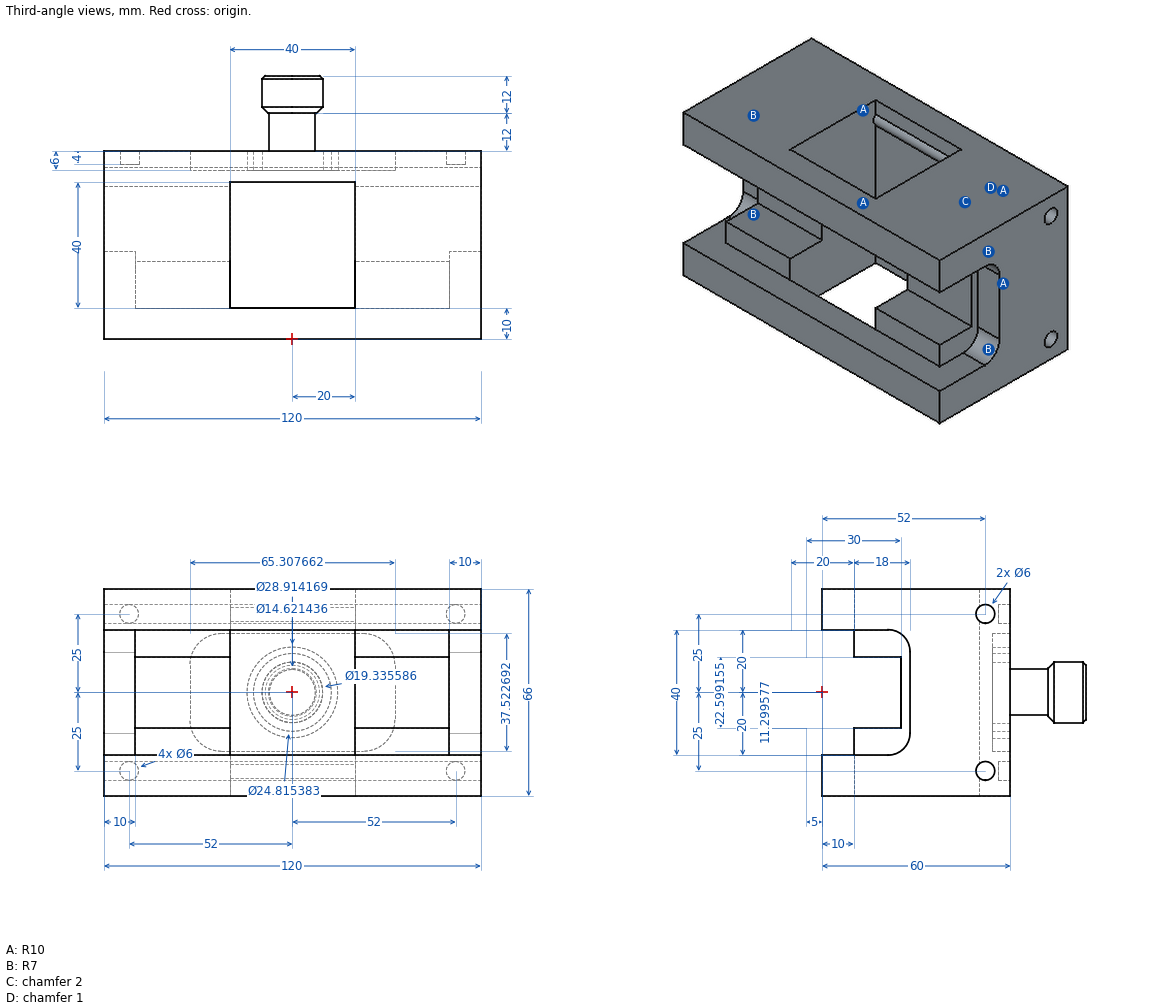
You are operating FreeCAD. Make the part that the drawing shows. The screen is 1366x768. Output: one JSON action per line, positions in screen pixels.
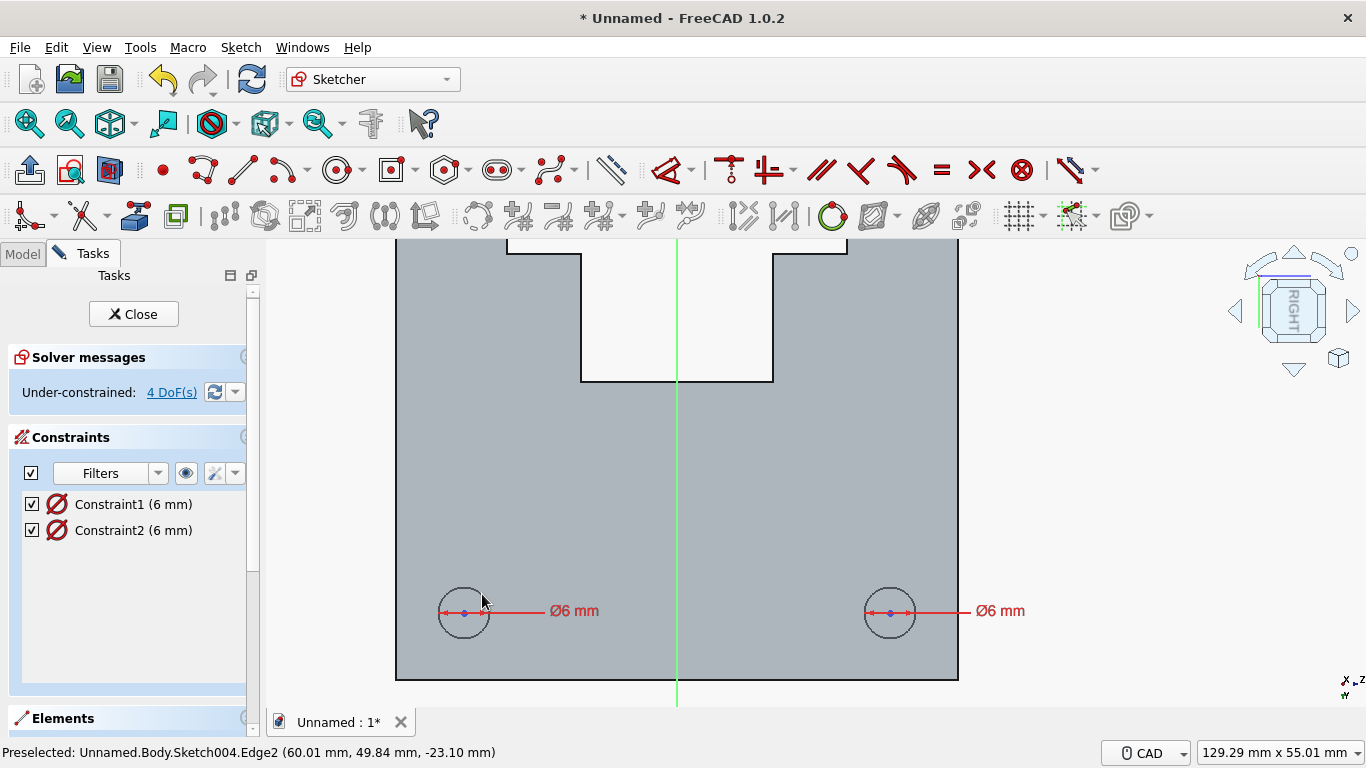
{"action": "left_click", "coordinate": [890, 613]}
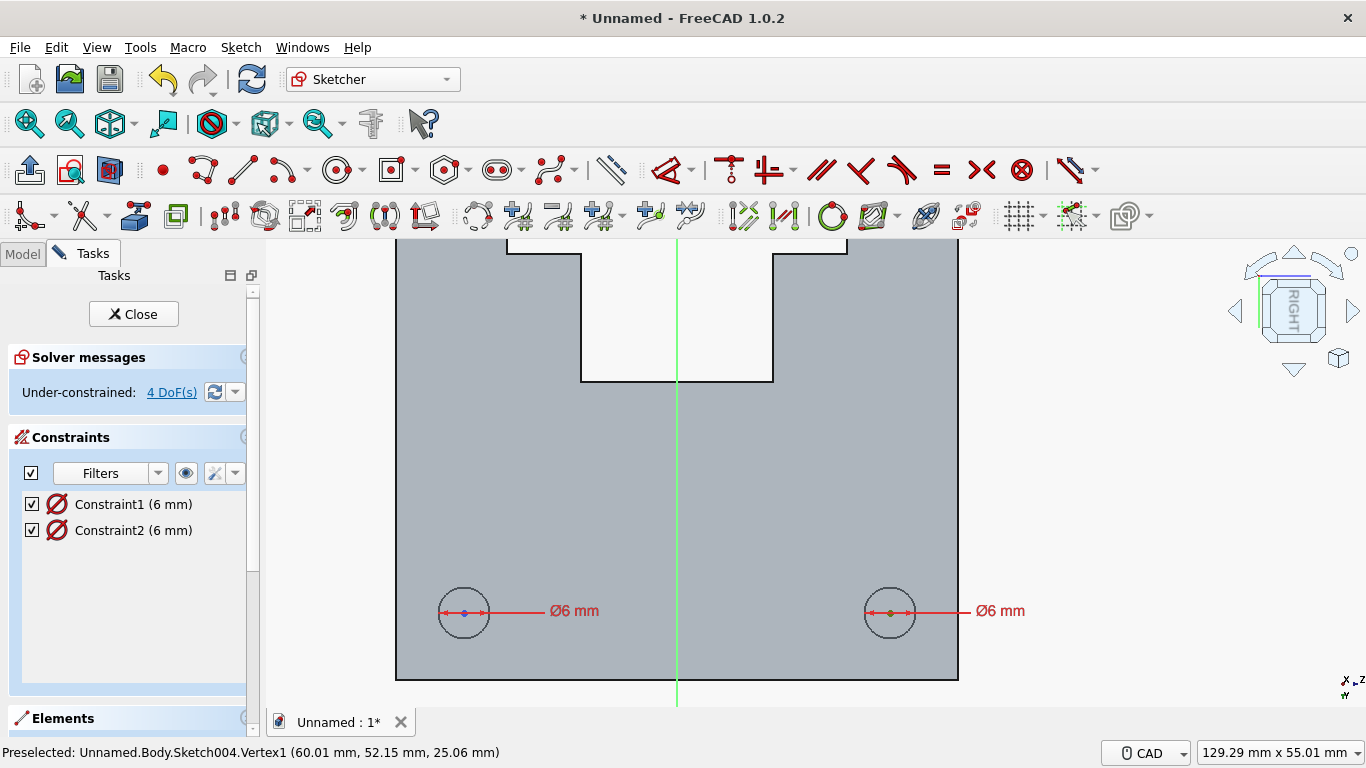
{"action": "left_click", "coordinate": [464, 613]}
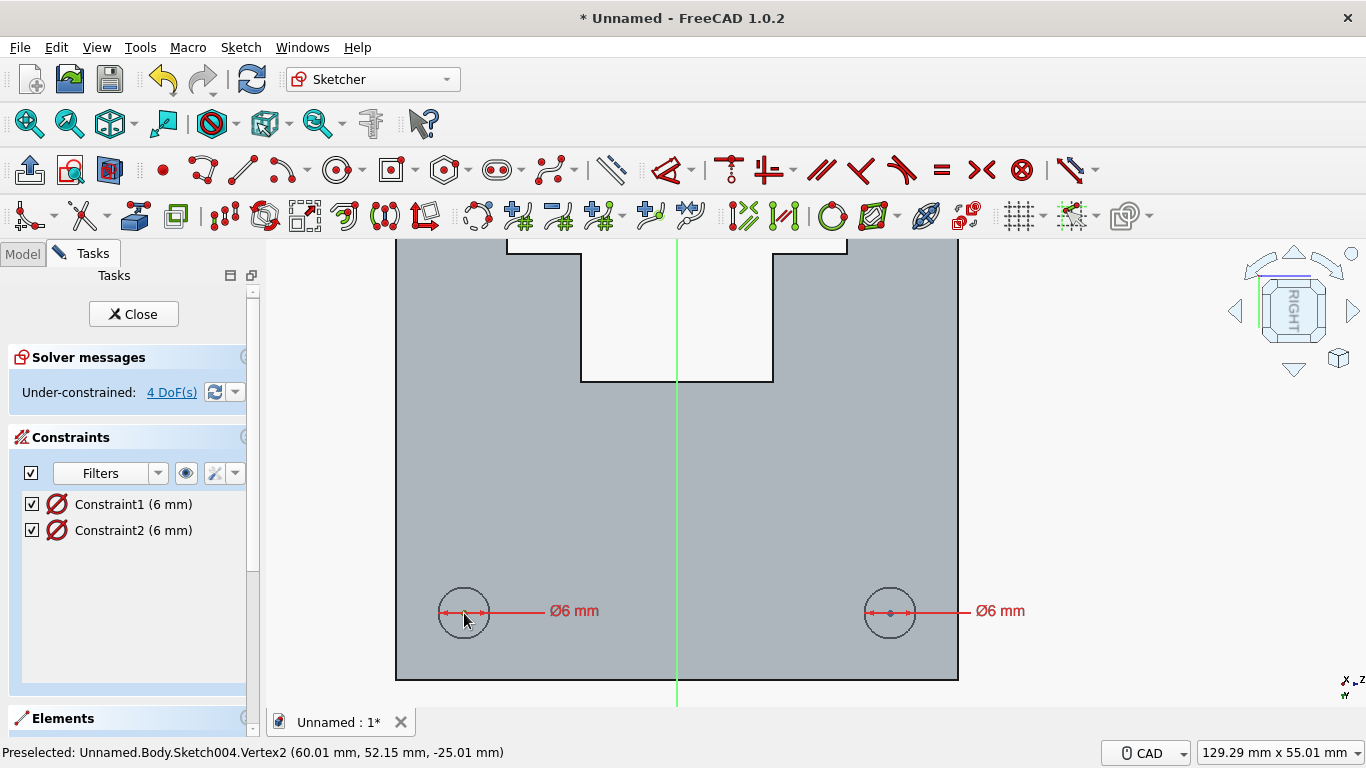
{"action": "key", "text": "h"}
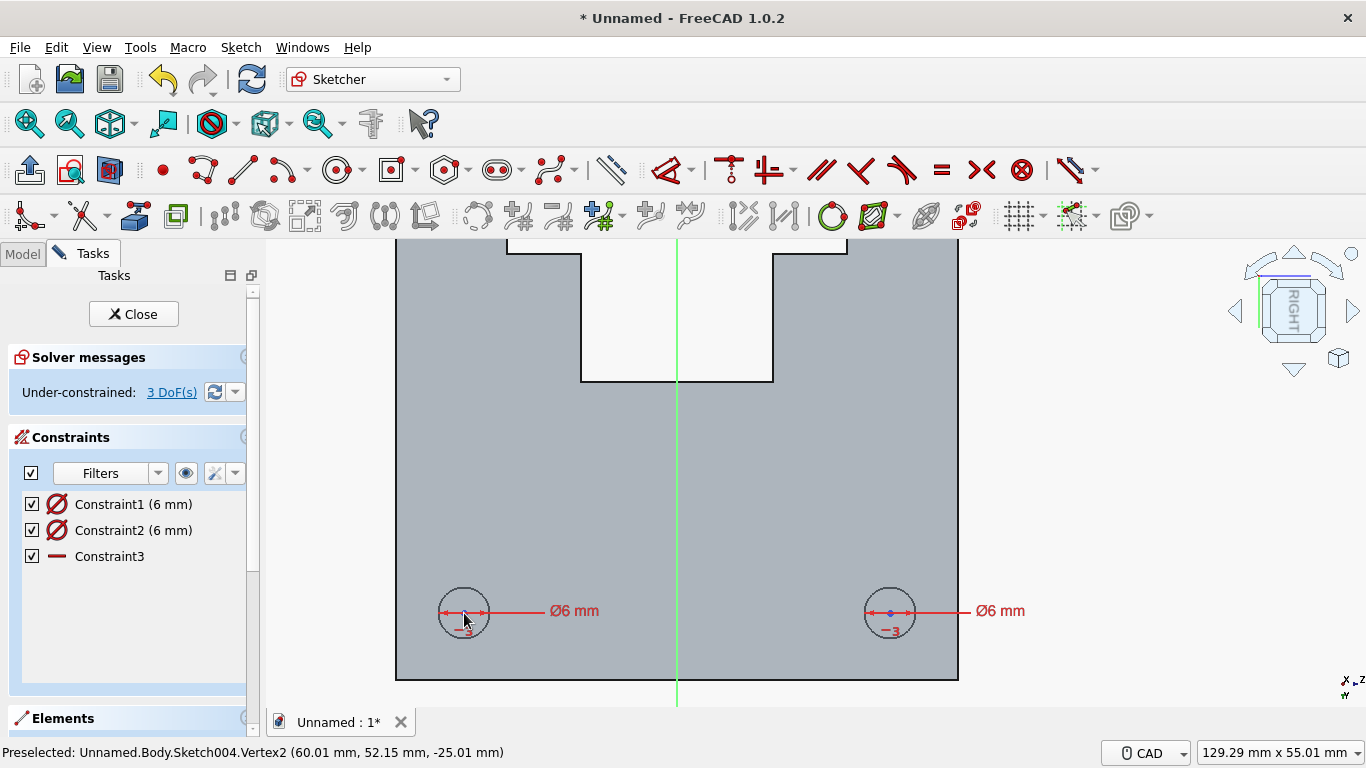
{"action": "left_click", "coordinate": [666, 170]}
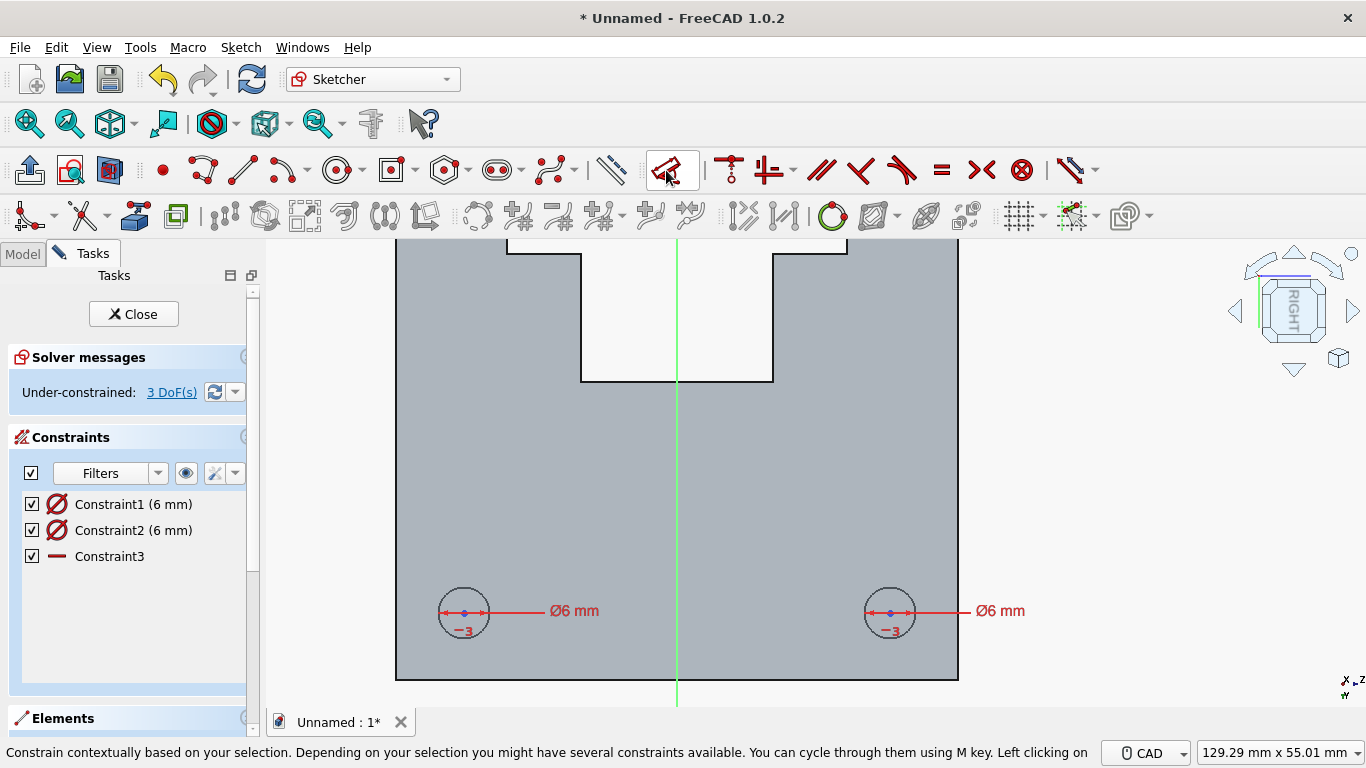
{"action": "left_click", "coordinate": [890, 613]}
{"action": "left_click", "coordinate": [783, 647]}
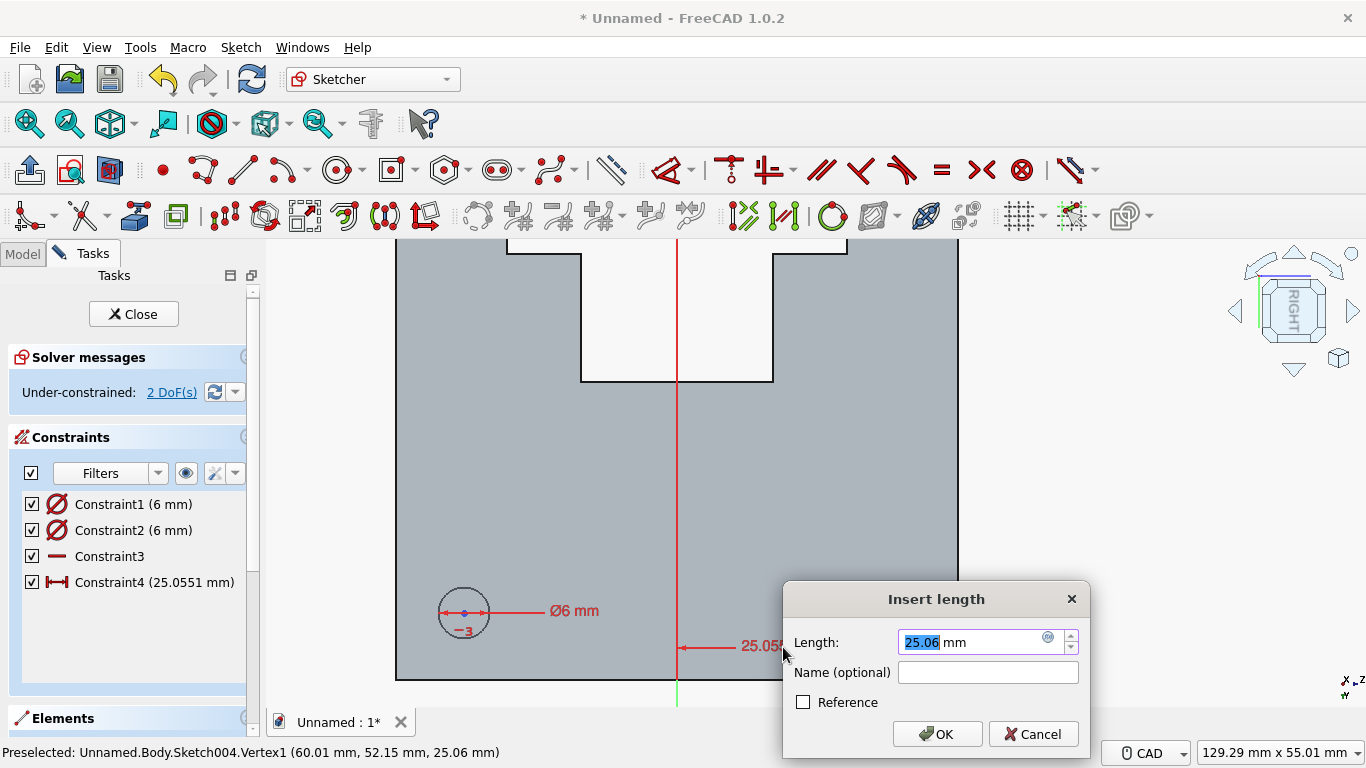
{"action": "type", "text": "25"}
{"action": "key", "text": "Return"}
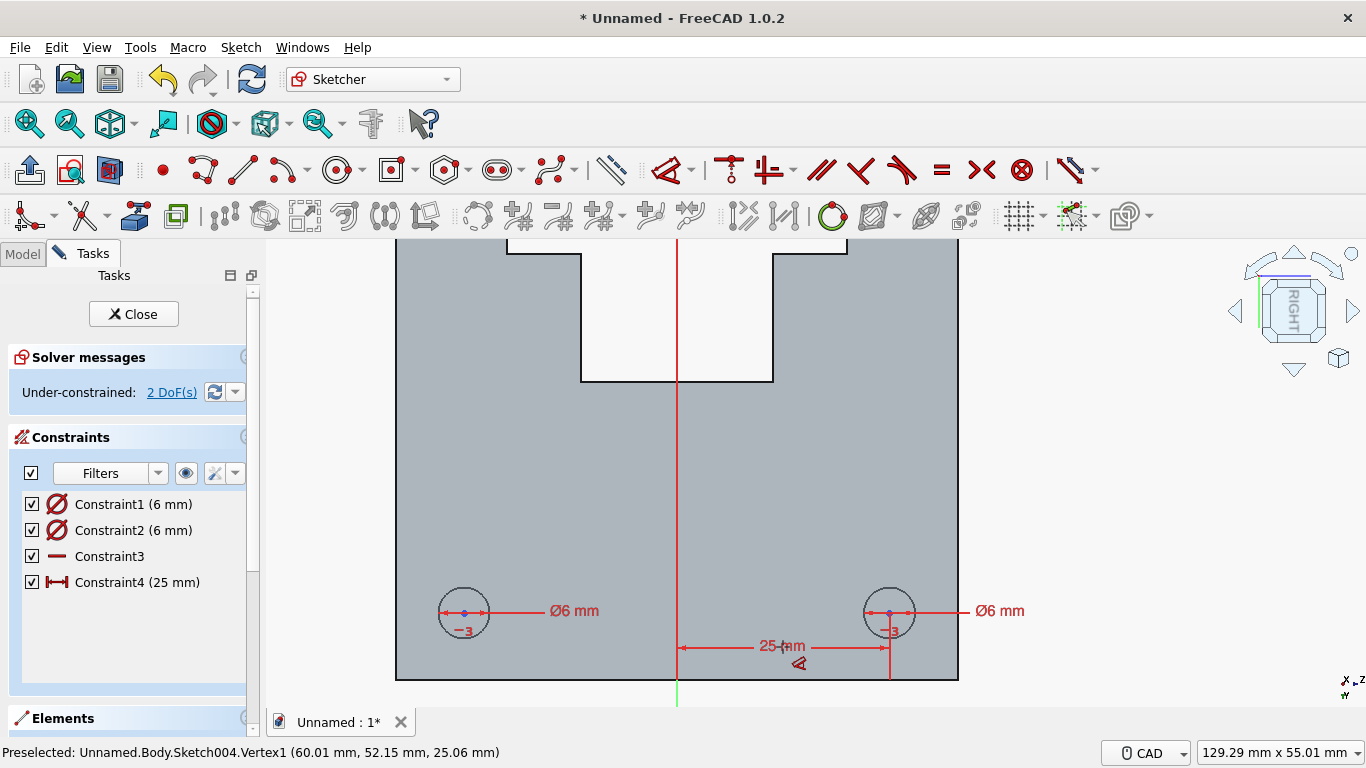
{"action": "left_click", "coordinate": [890, 613]}
{"action": "left_click", "coordinate": [924, 440]}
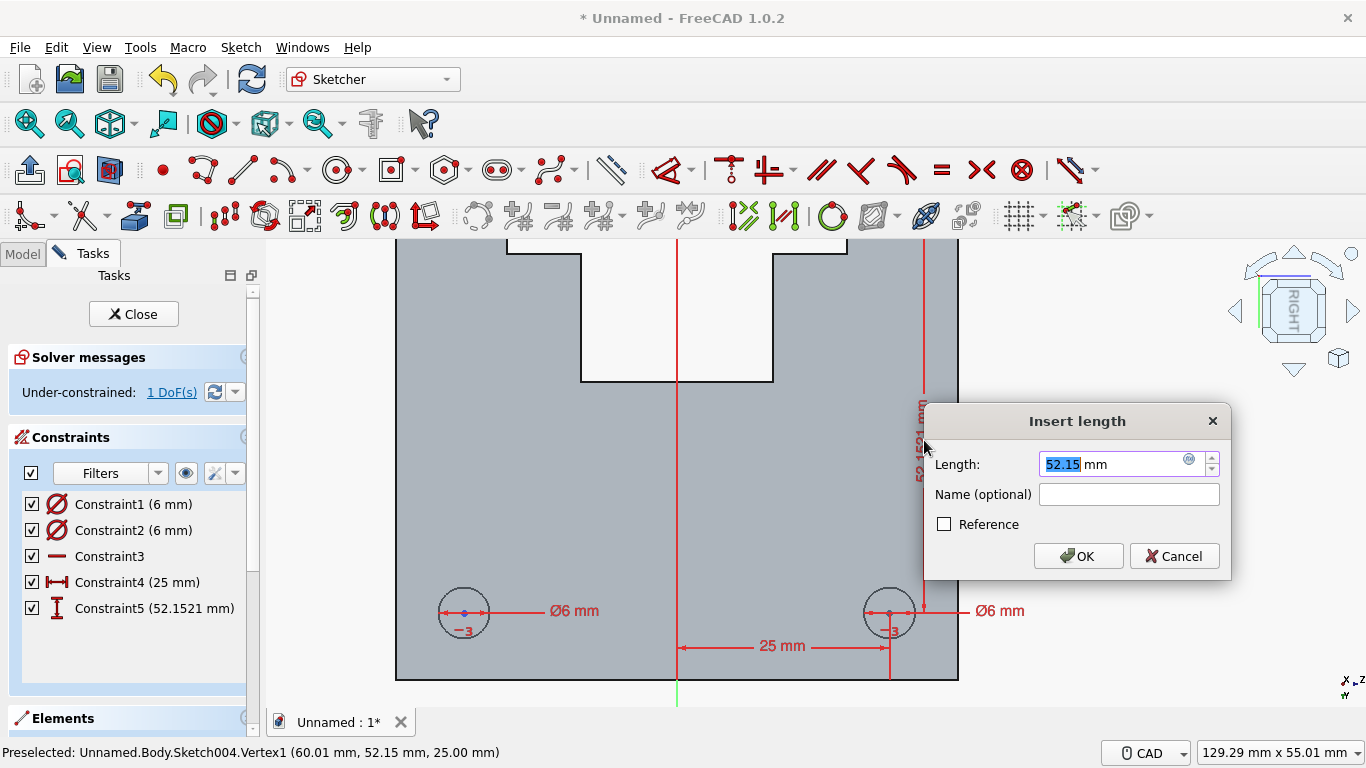
{"action": "type", "text": "52"}
{"action": "key", "text": "Return"}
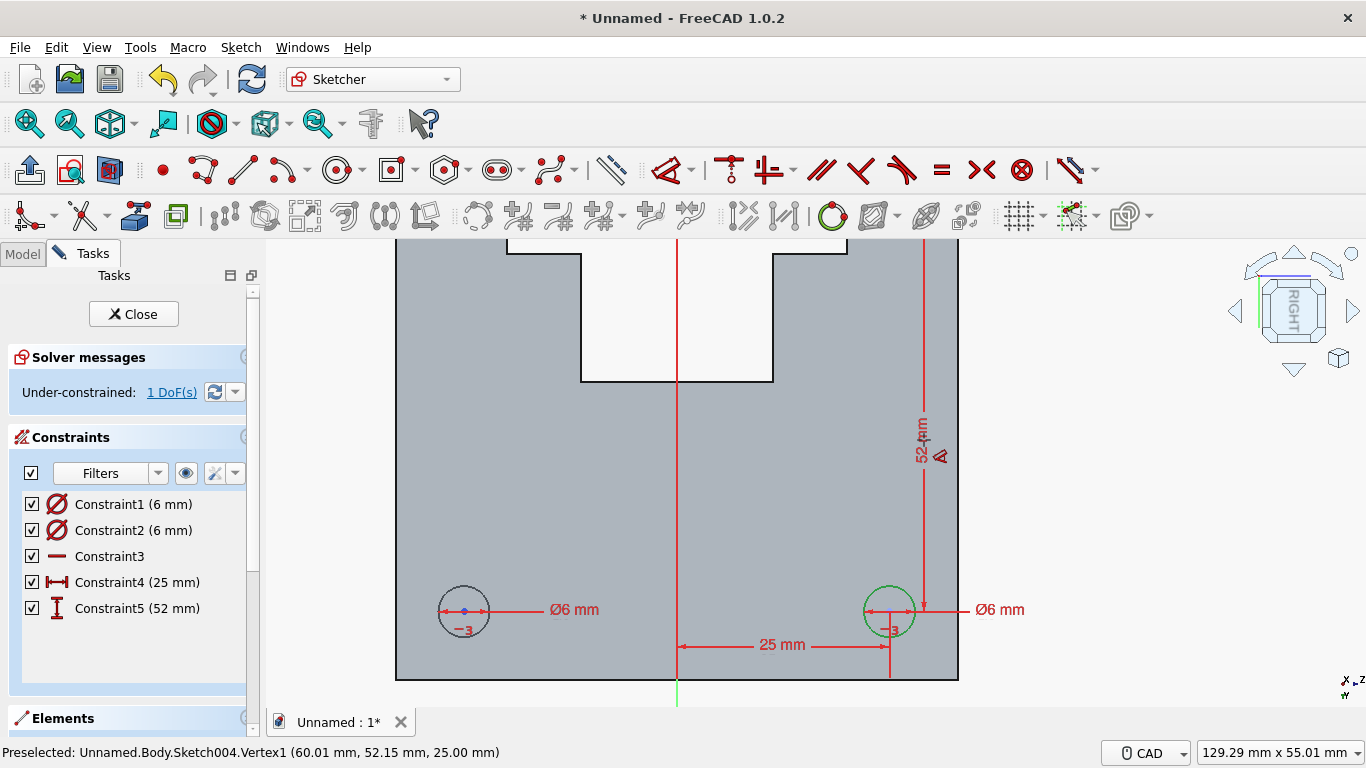
{"action": "left_click", "coordinate": [464, 612]}
{"action": "left_click", "coordinate": [570, 646]}